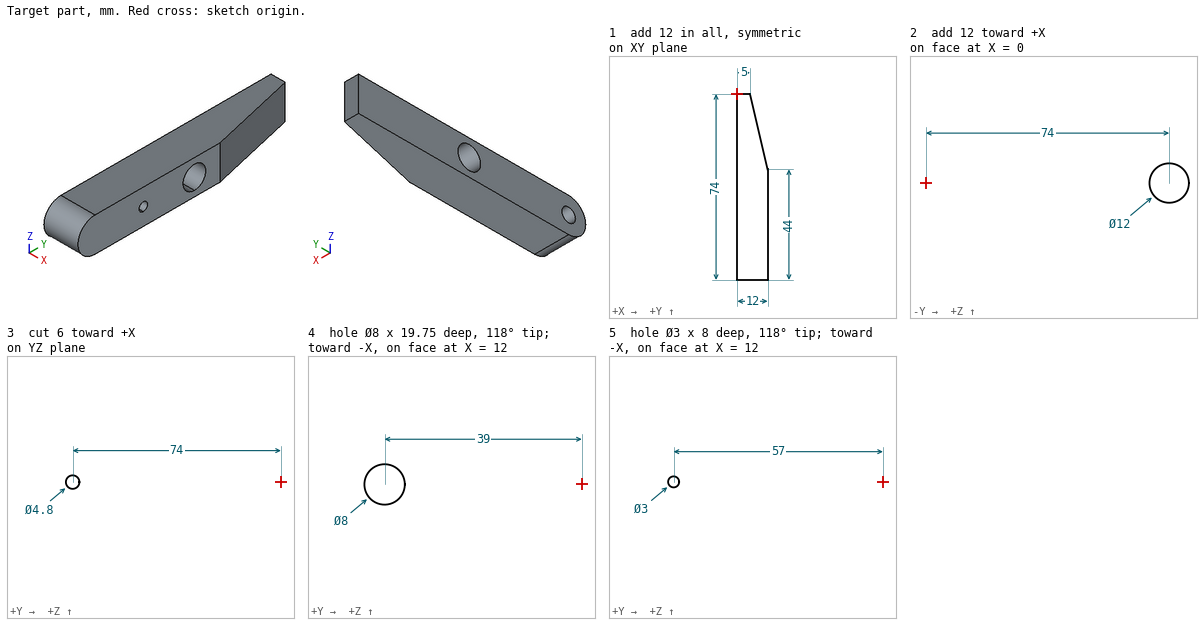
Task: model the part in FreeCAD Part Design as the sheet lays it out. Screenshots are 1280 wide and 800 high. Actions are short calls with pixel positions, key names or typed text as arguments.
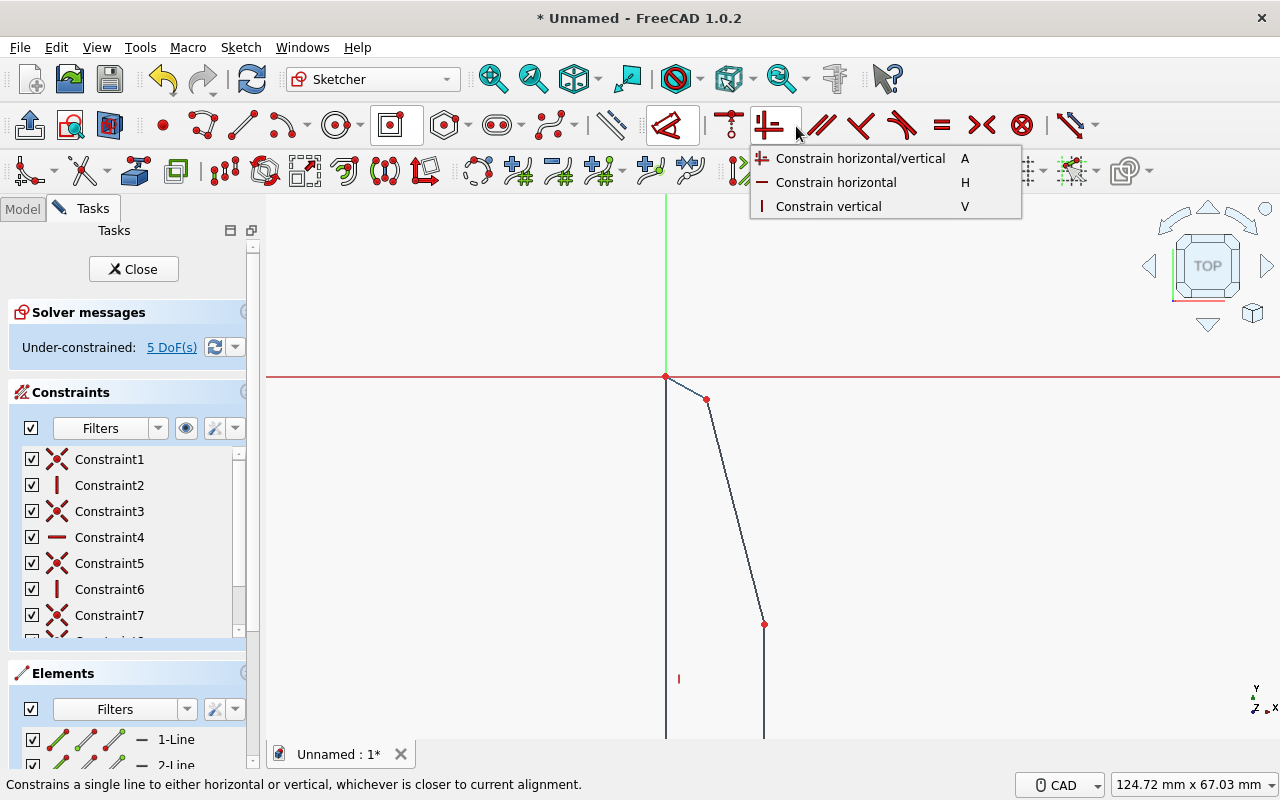
click(886, 182)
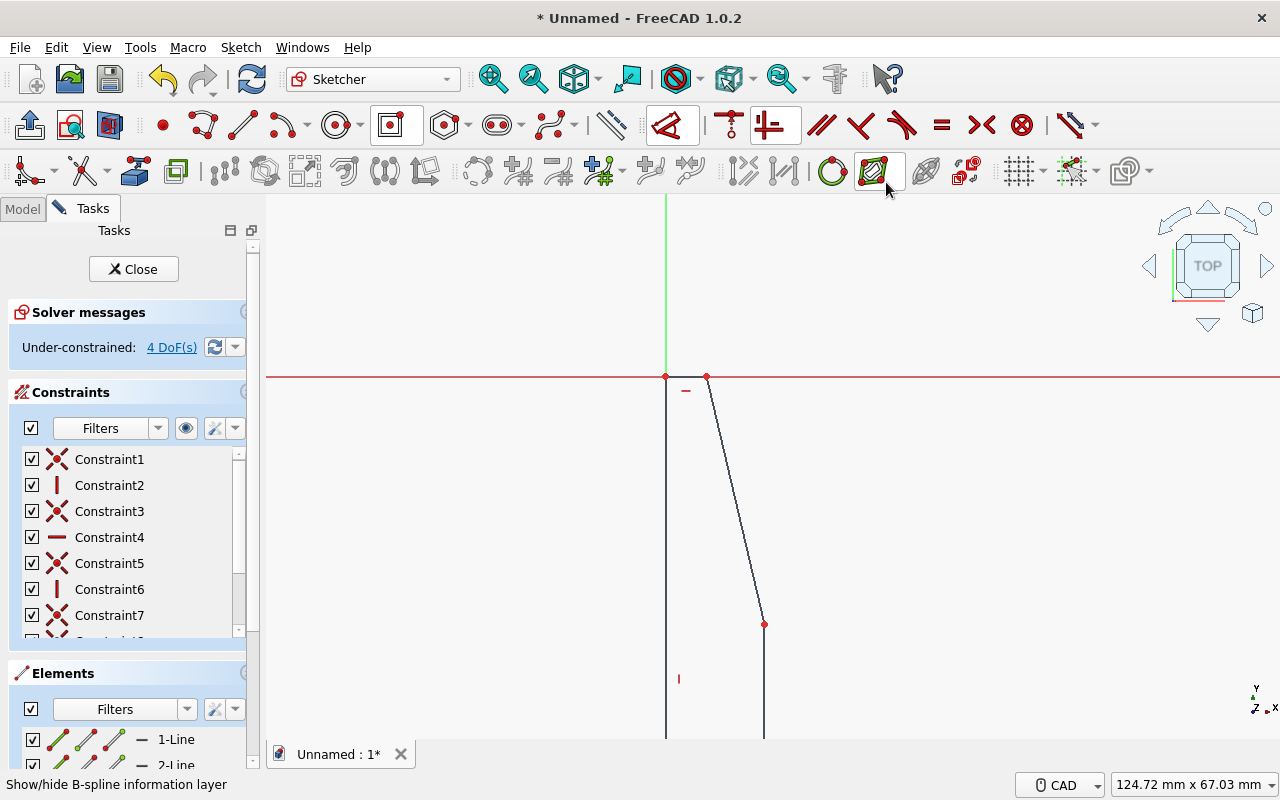
click(666, 126)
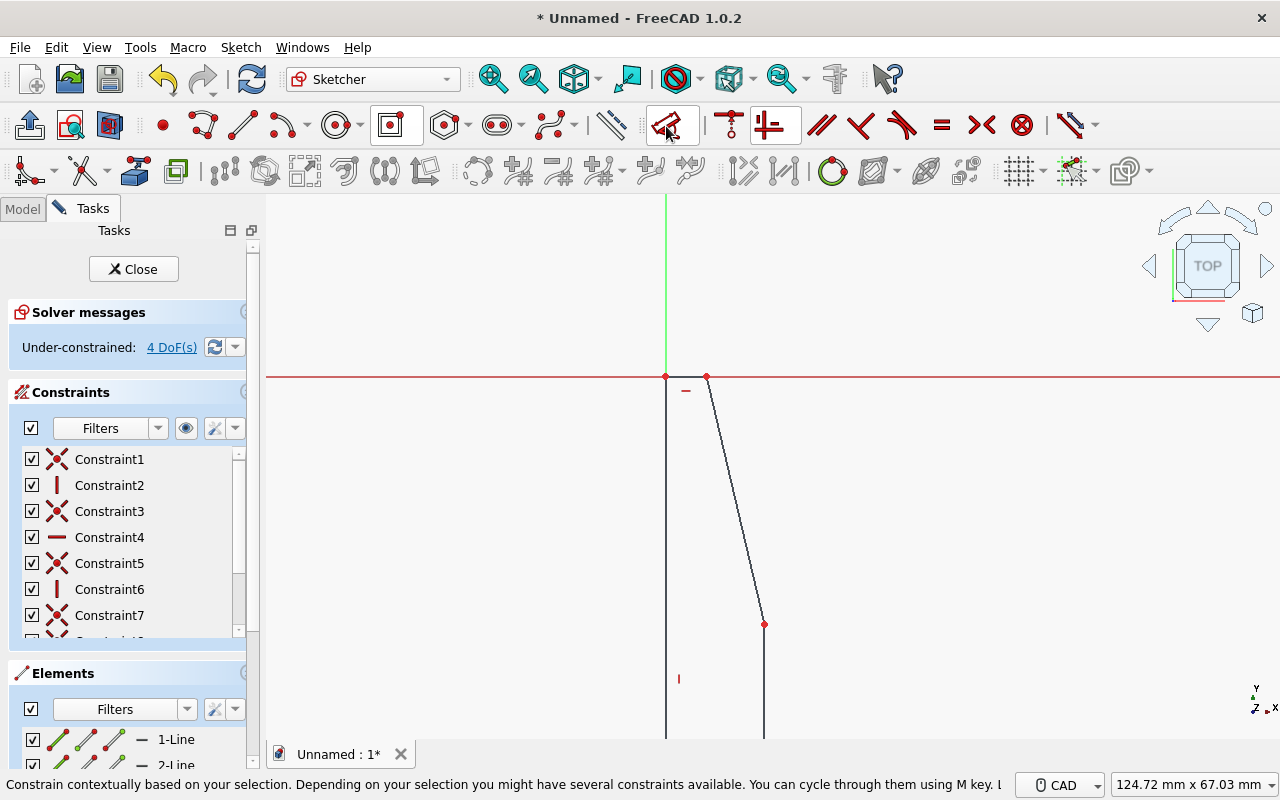
click(694, 377)
click(686, 343)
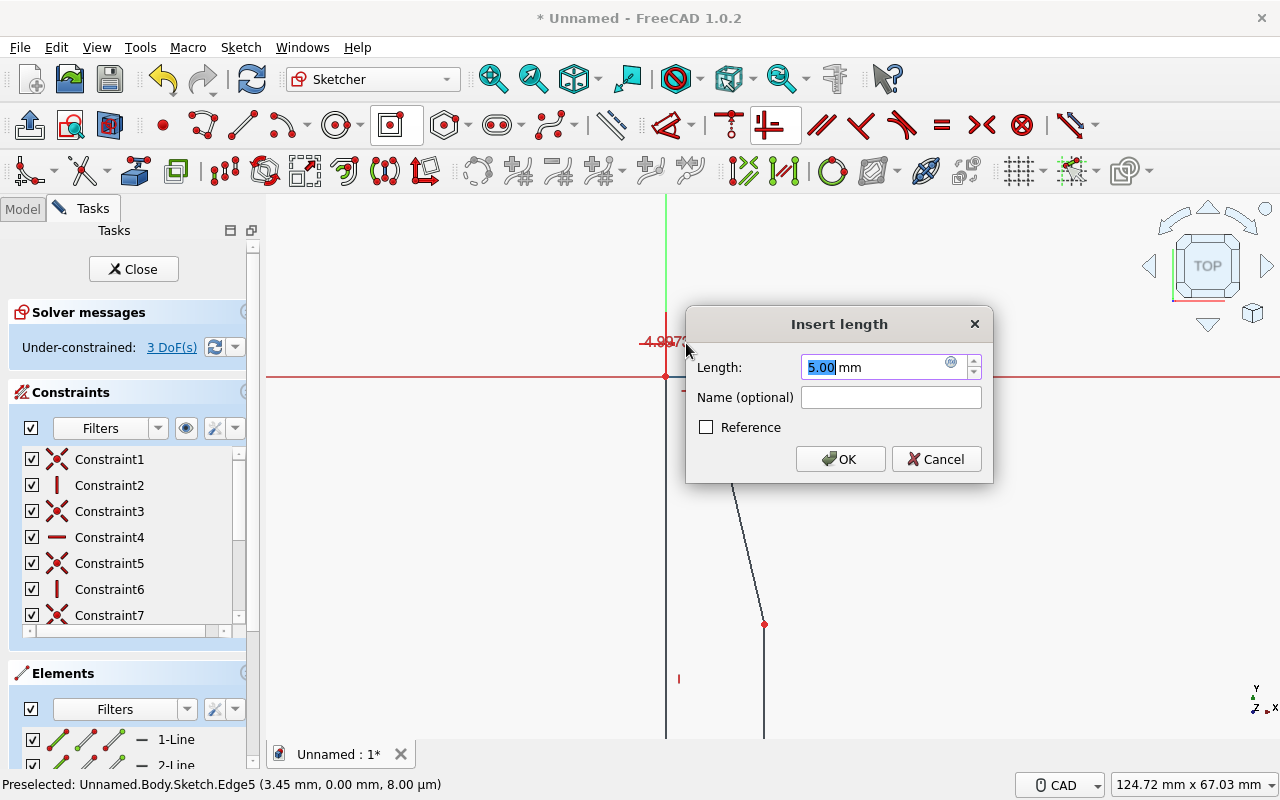
text(5)
key(Return)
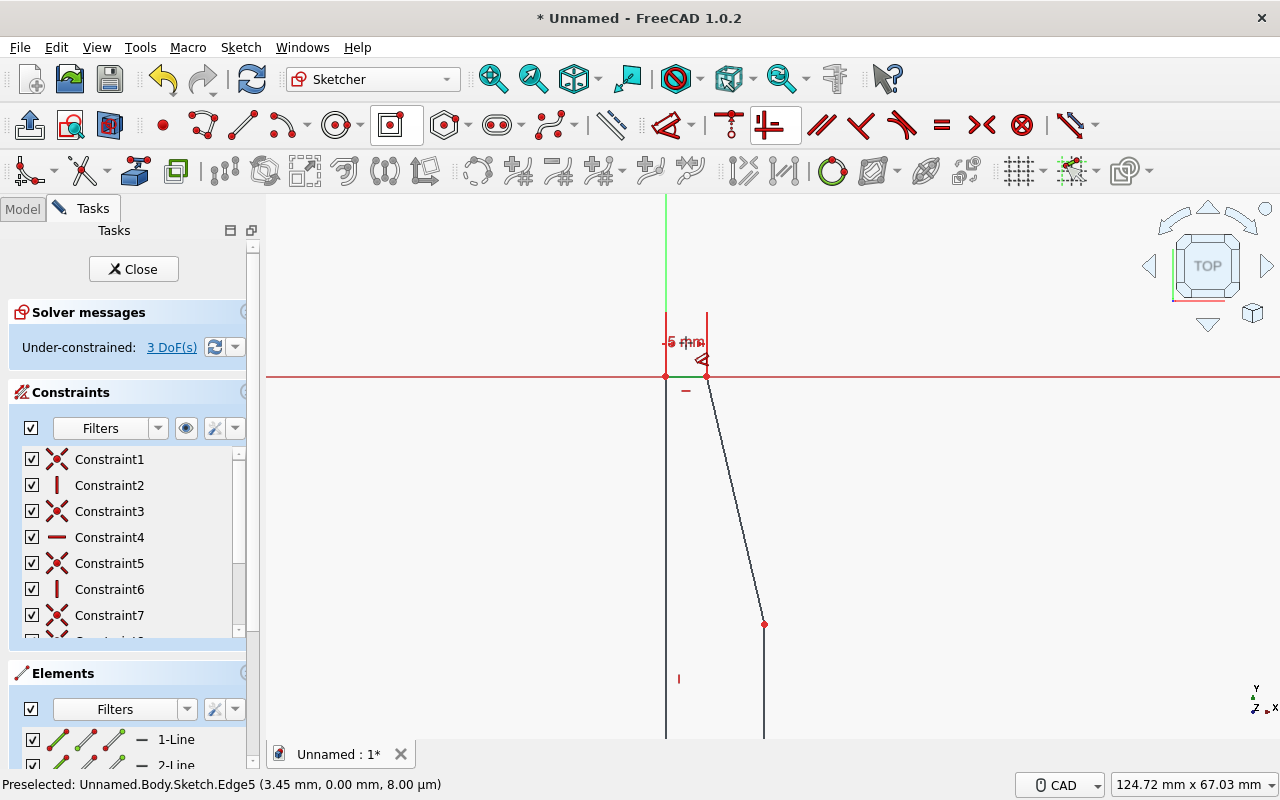
click(666, 558)
click(632, 544)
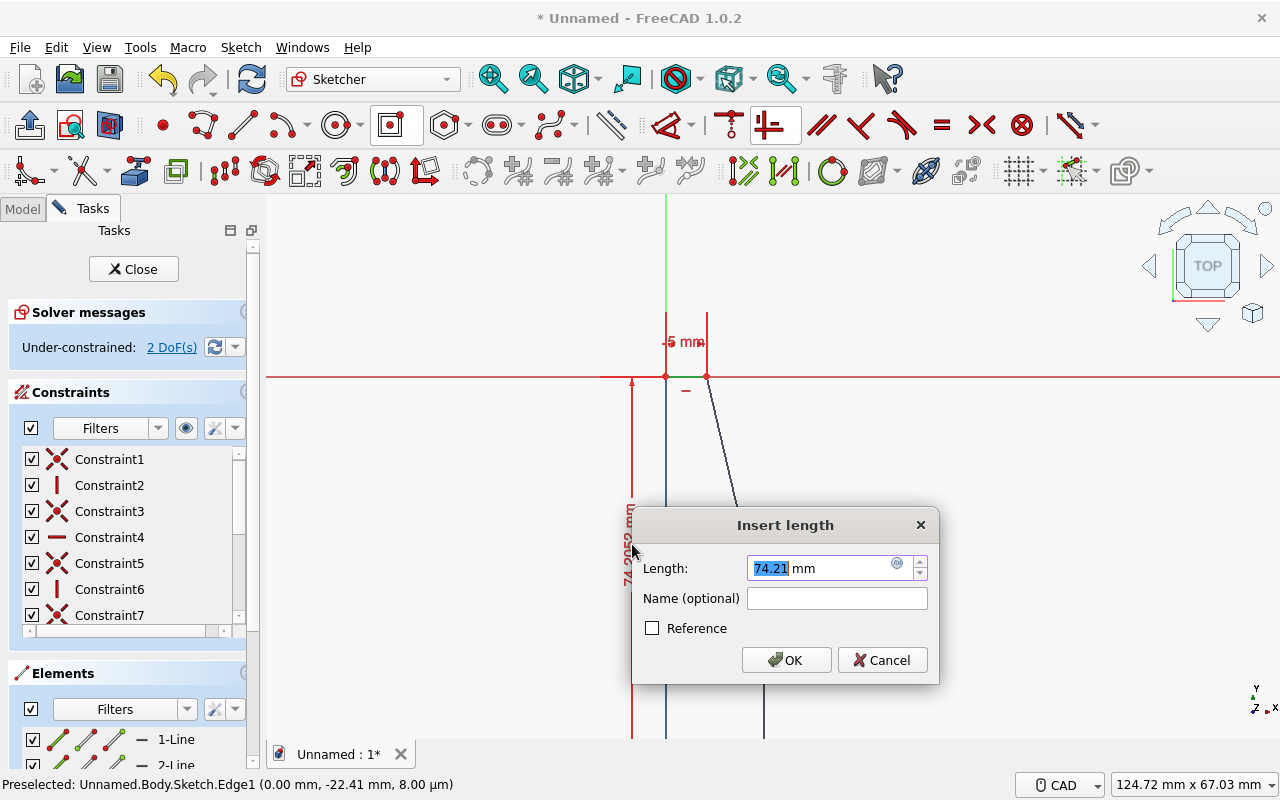
text(74)
key(Return)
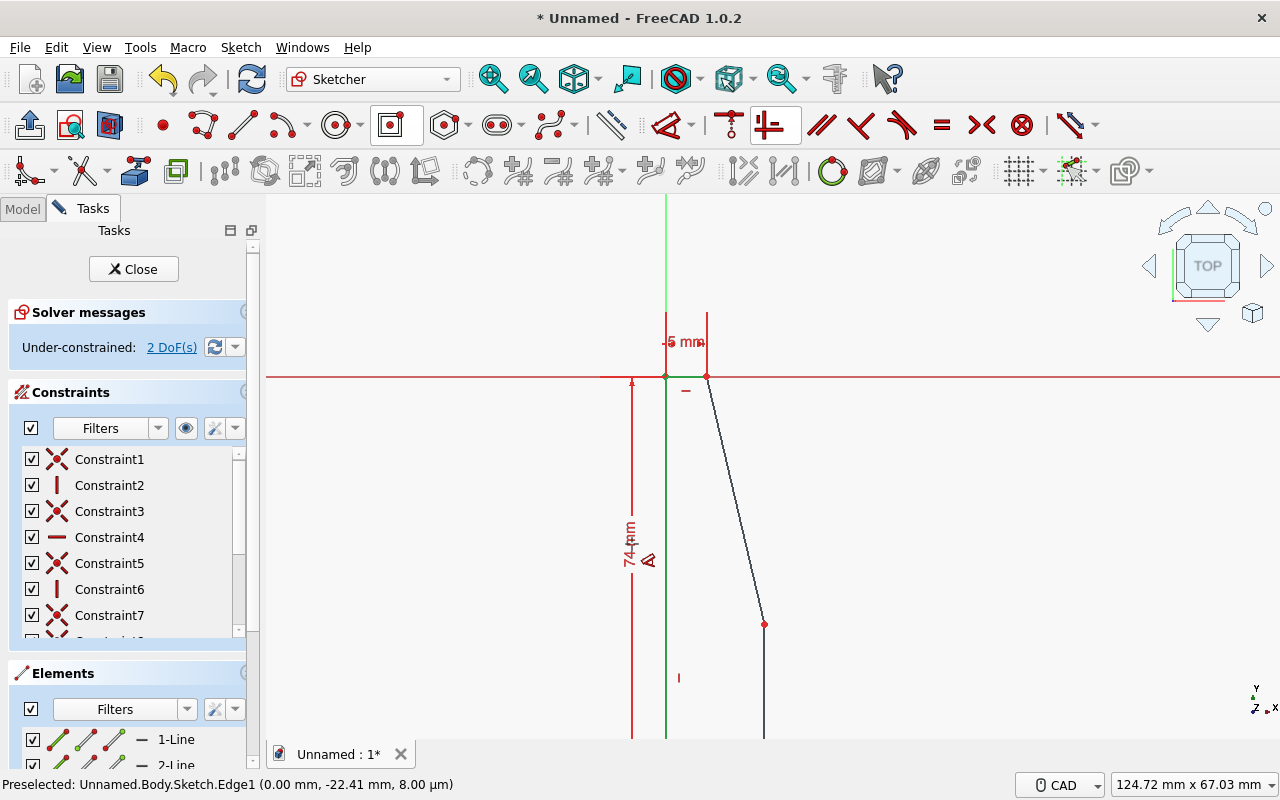
scroll(692, 222, down, 3)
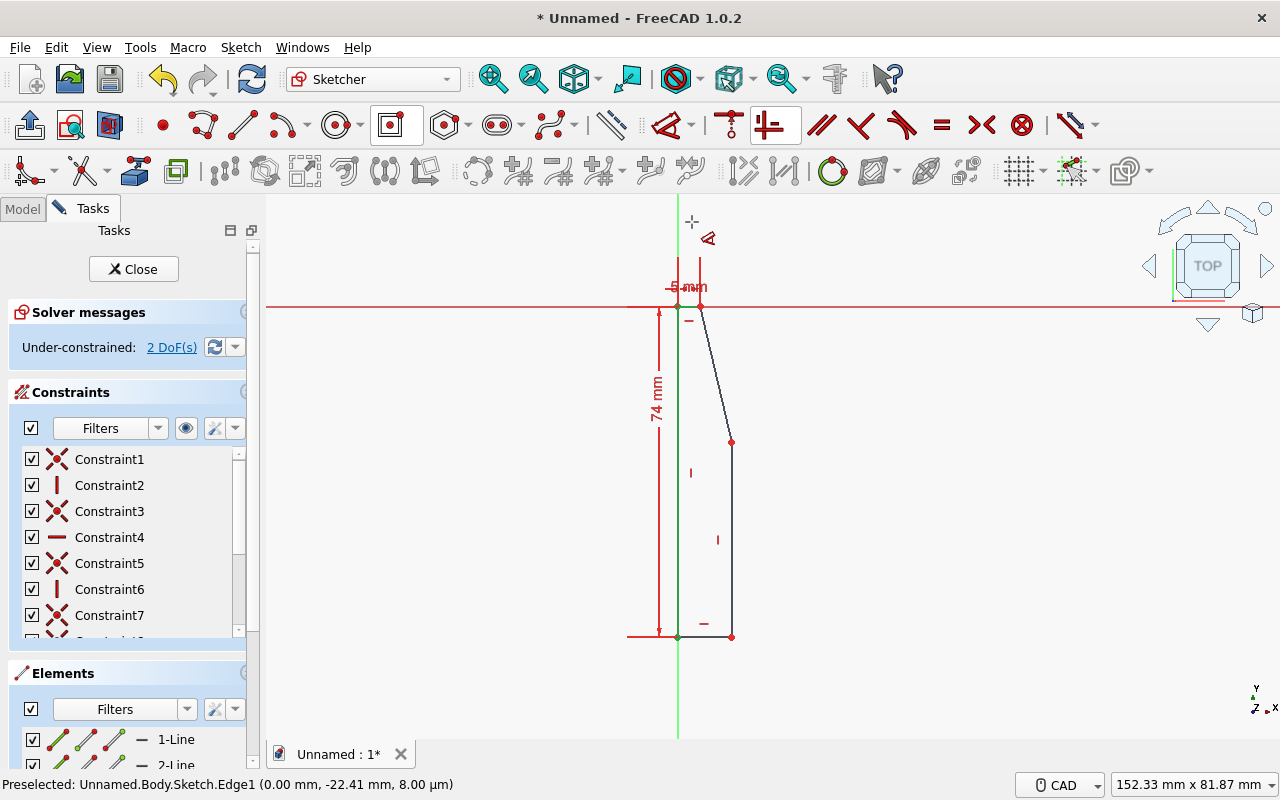
click(694, 637)
click(705, 671)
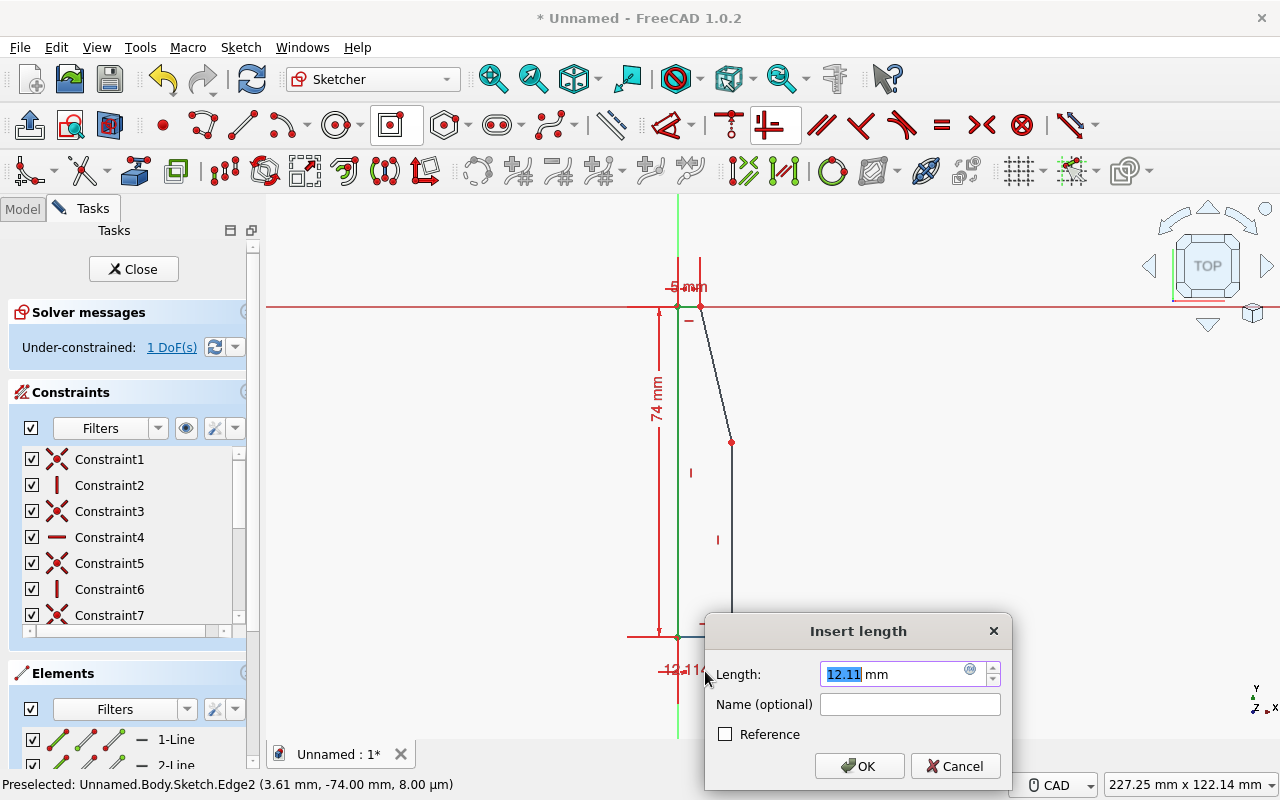
text(12)
key(Return)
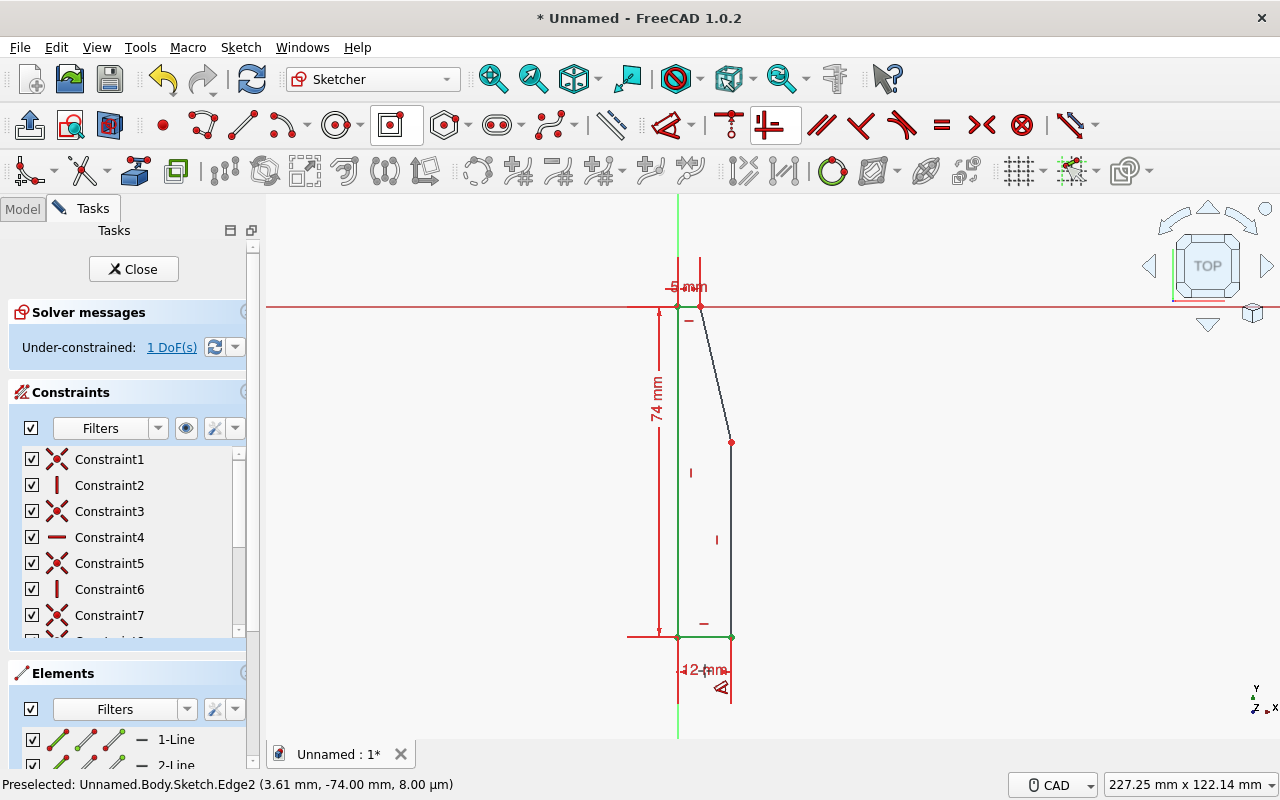
click(731, 579)
click(765, 540)